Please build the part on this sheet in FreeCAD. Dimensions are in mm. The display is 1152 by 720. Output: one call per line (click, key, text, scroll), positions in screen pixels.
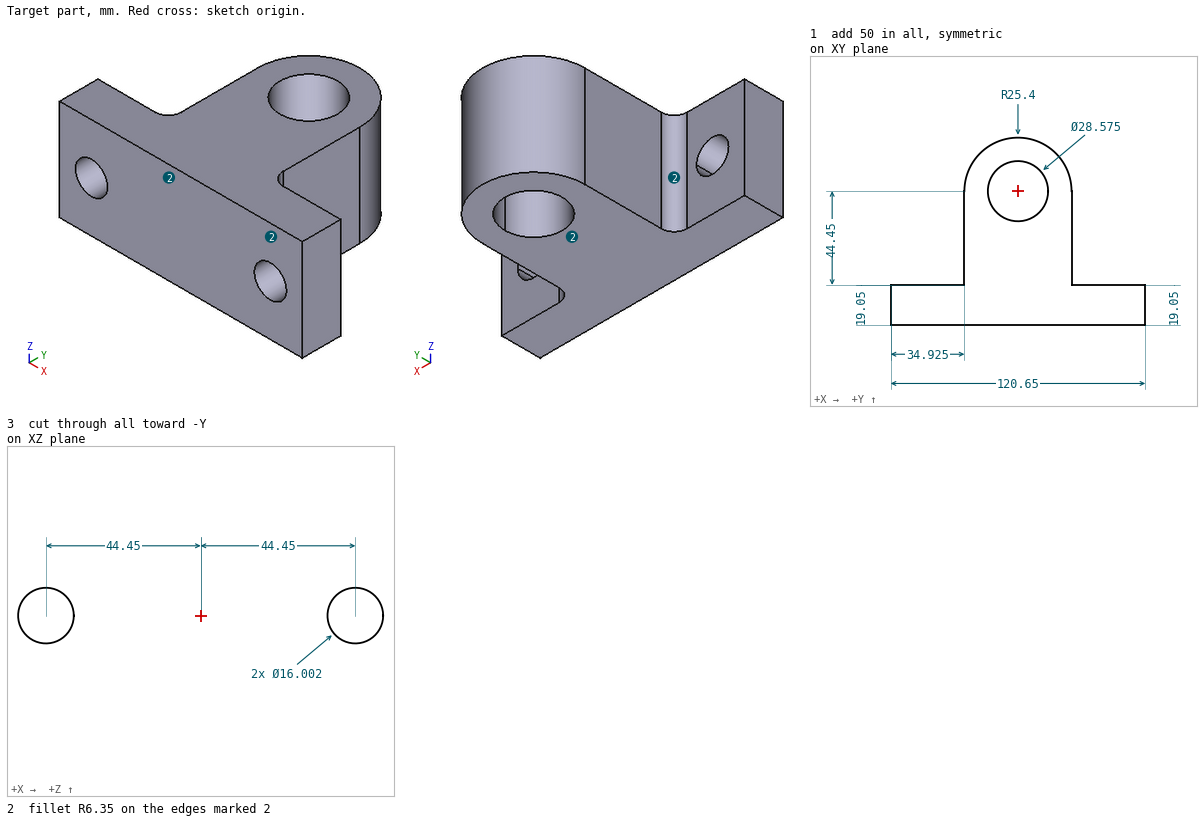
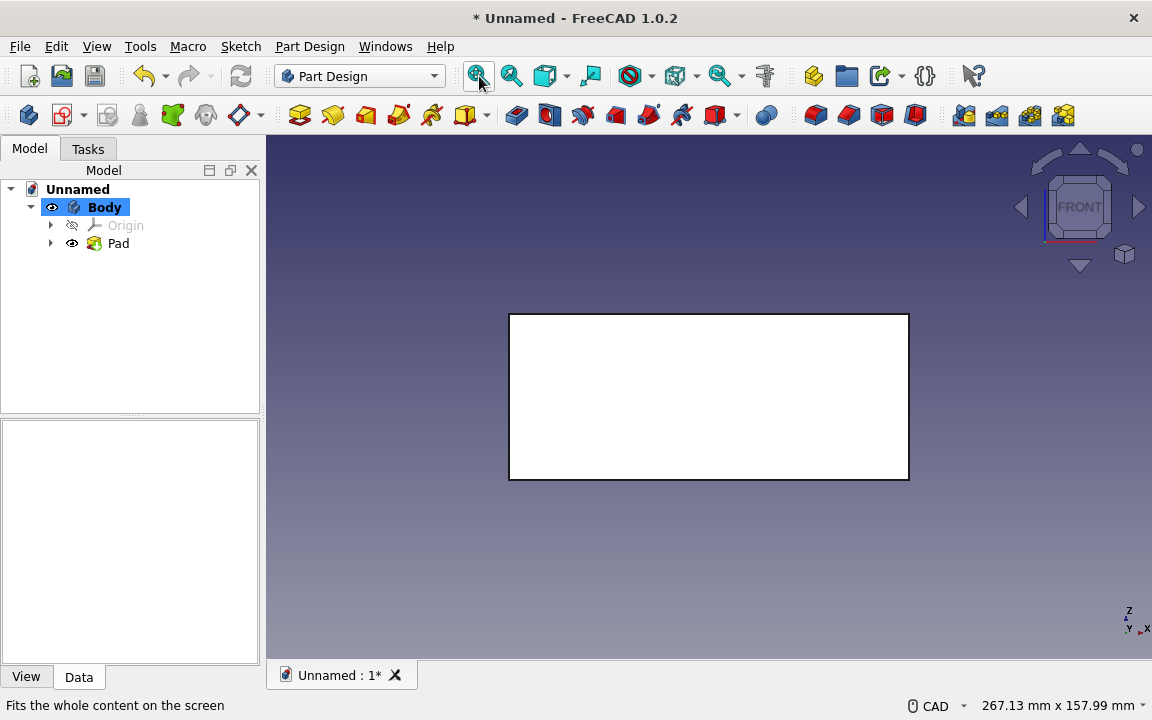
key(3)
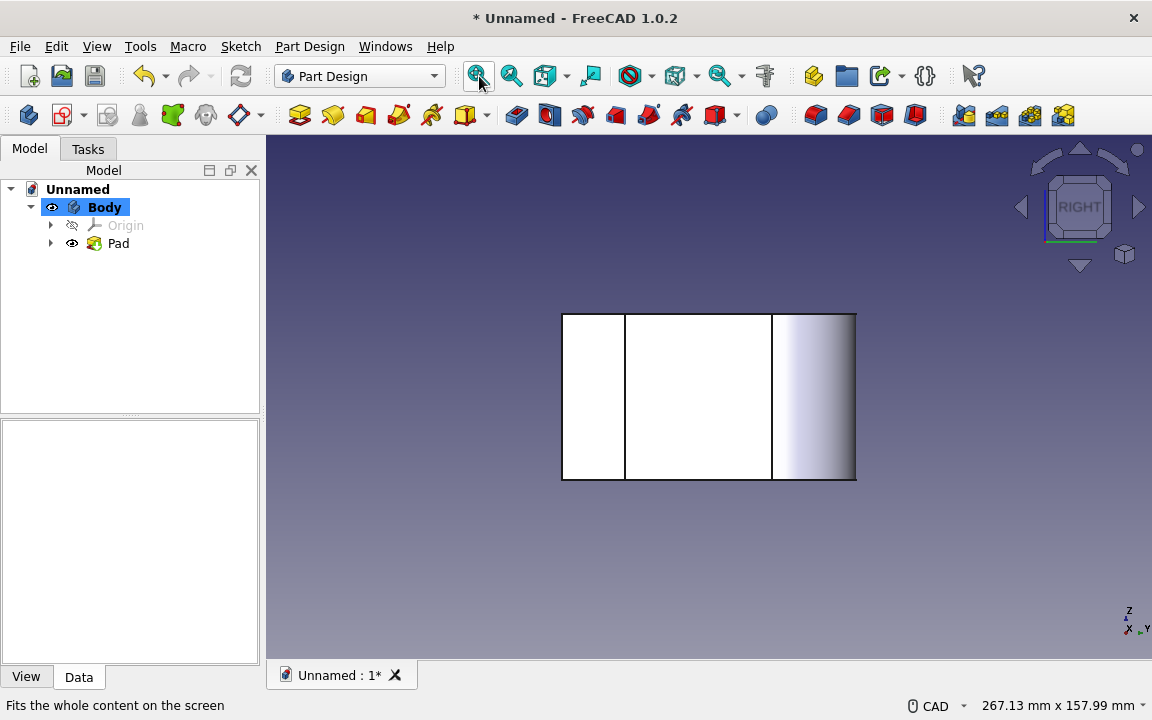
click(479, 76)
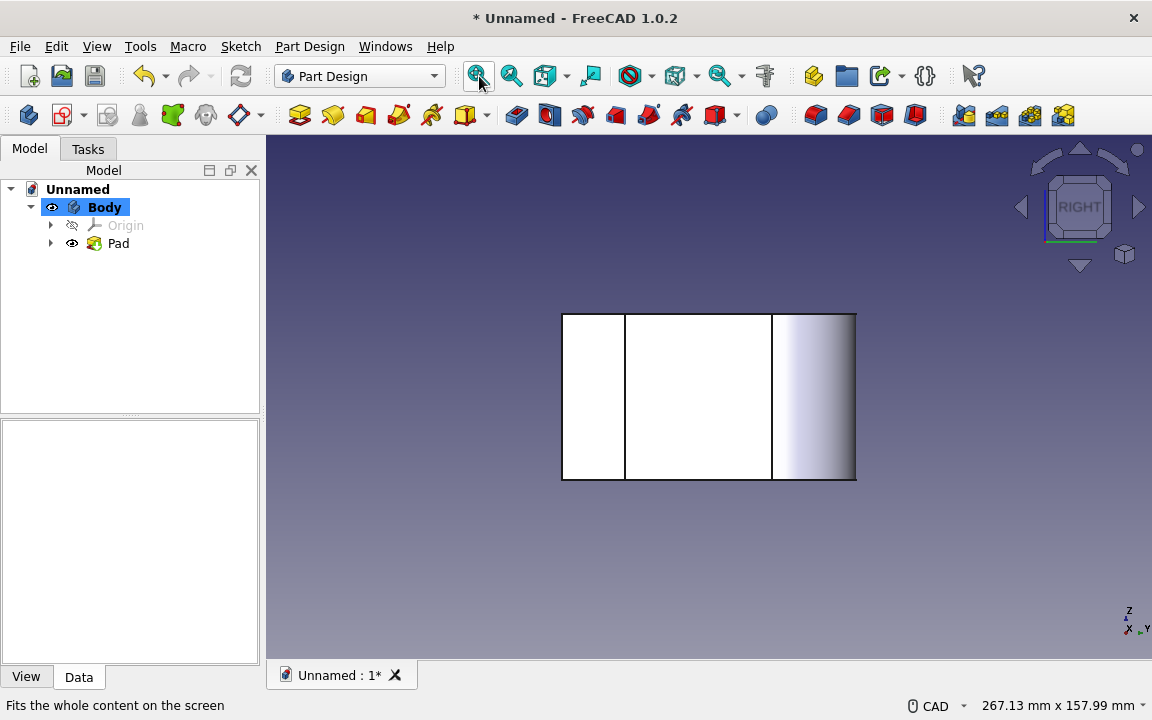
key(5)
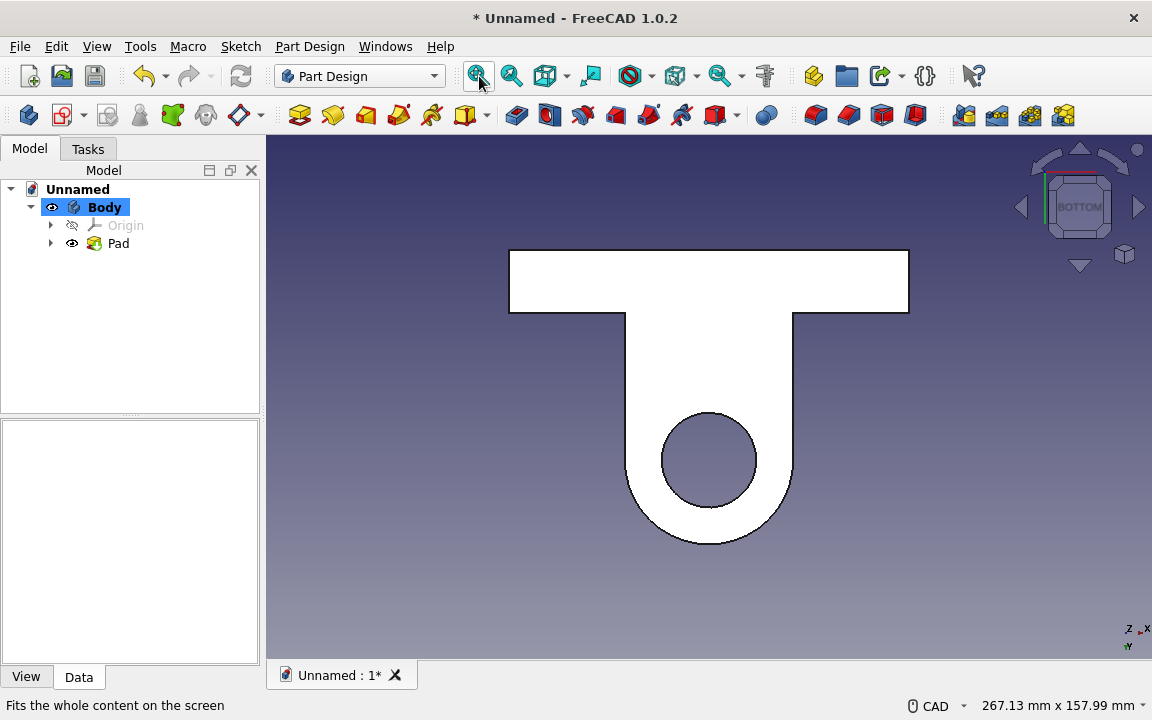
key(4)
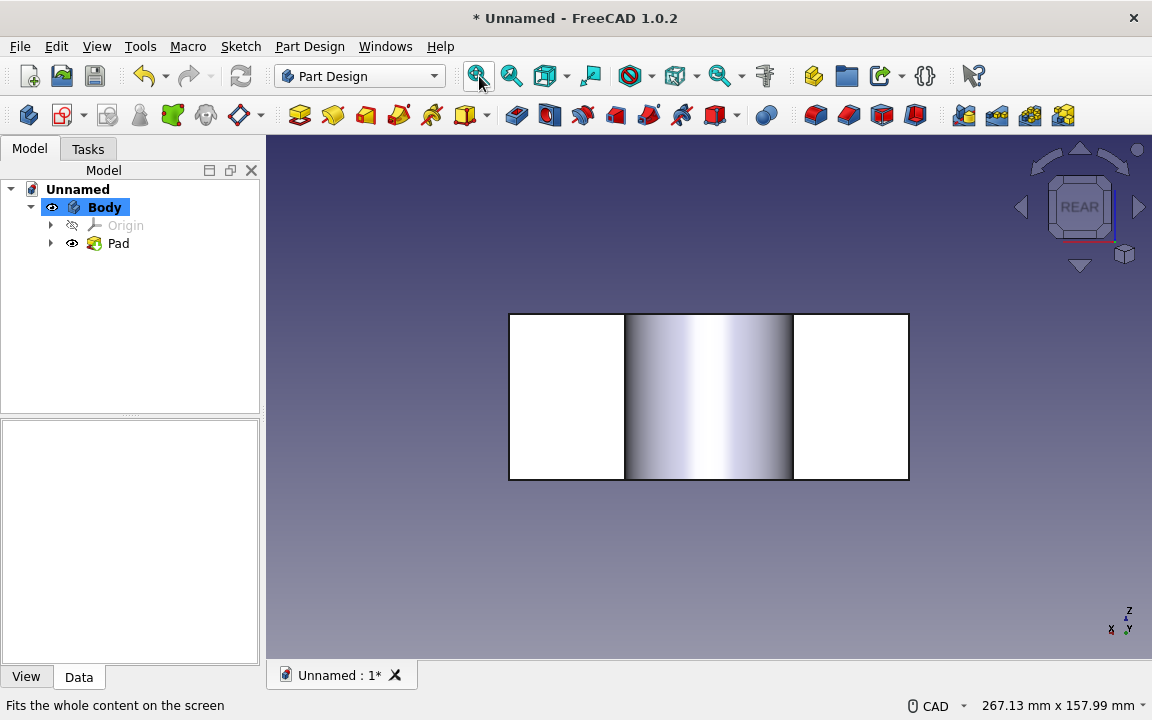
key(6)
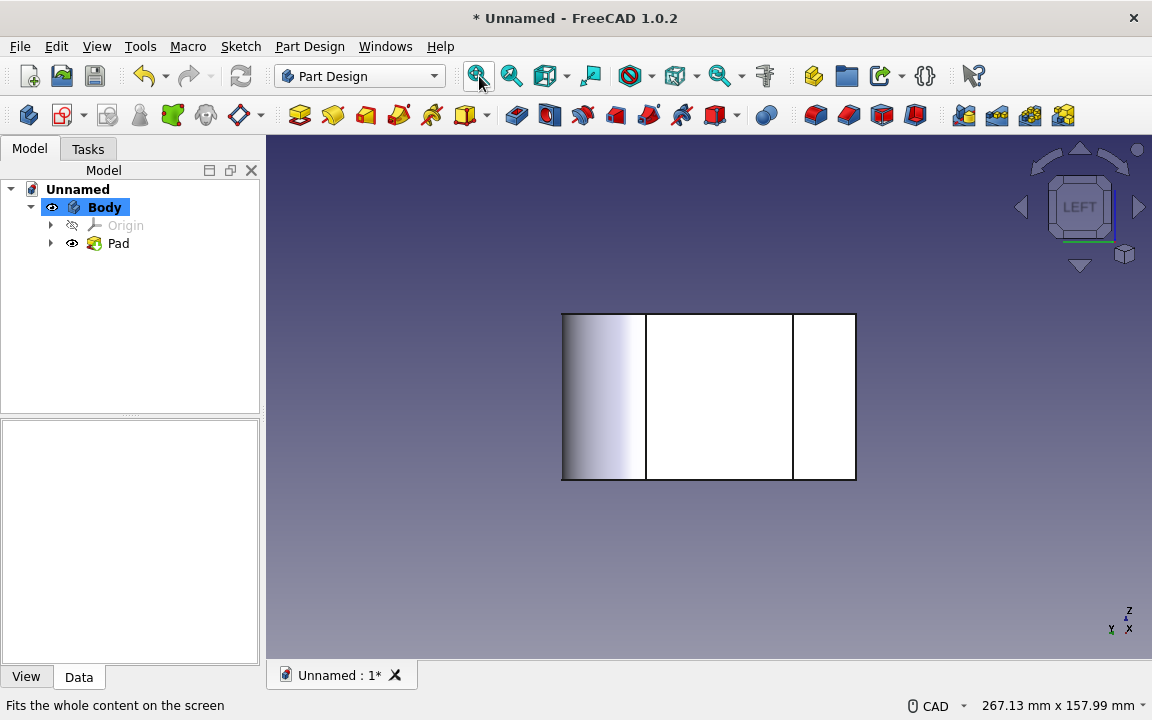
click(479, 76)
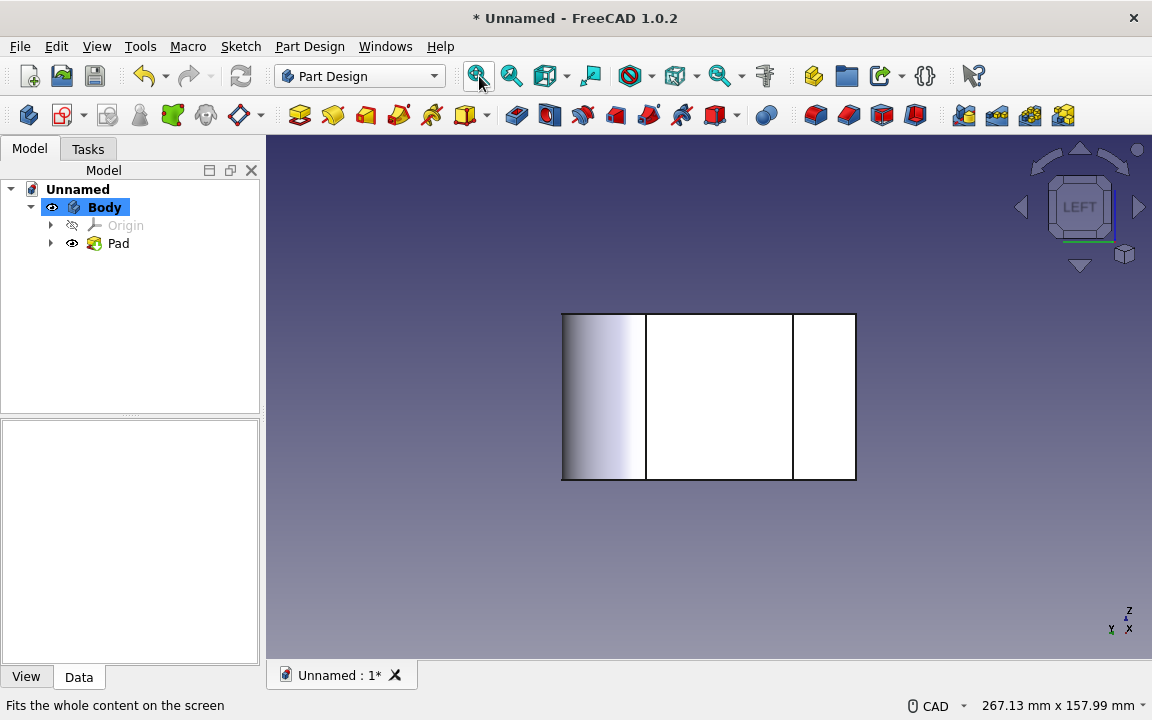
key(v)
key(3)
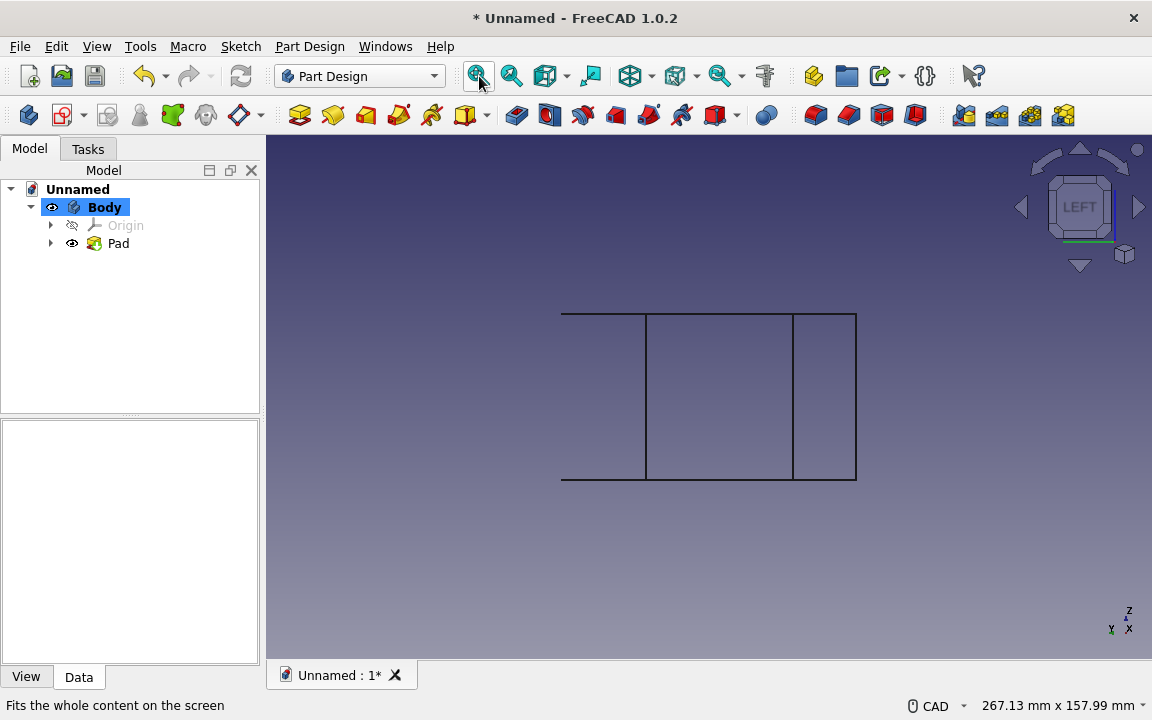
key(0)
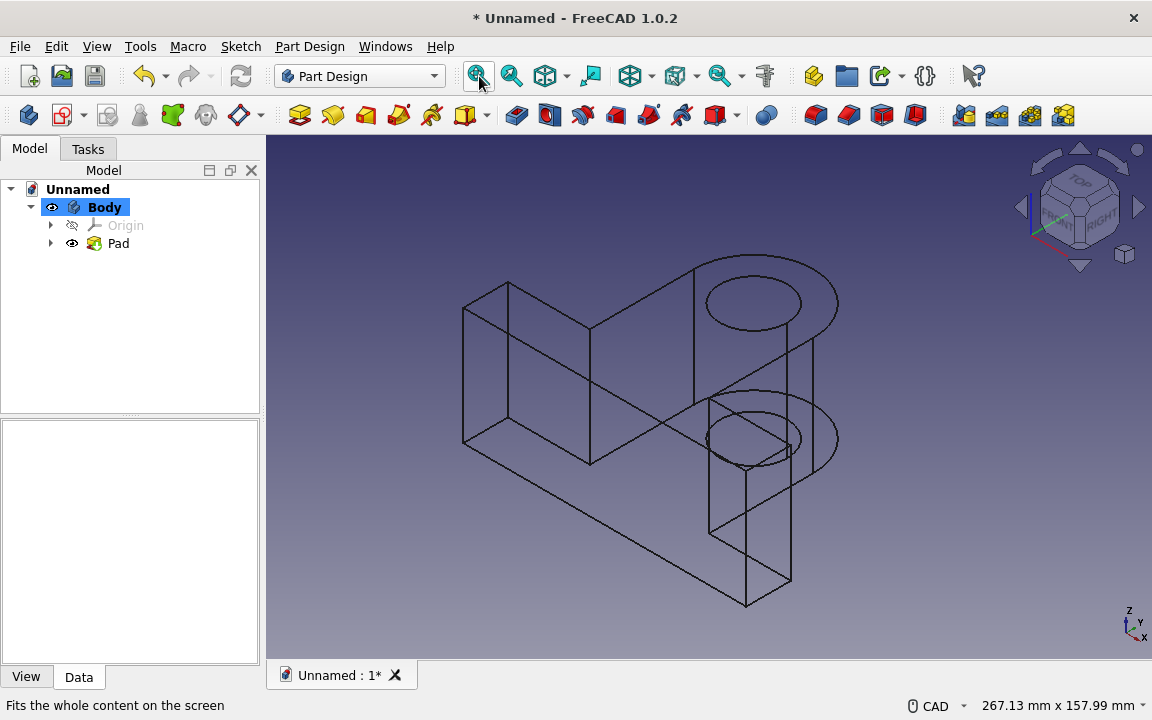
click(709, 465)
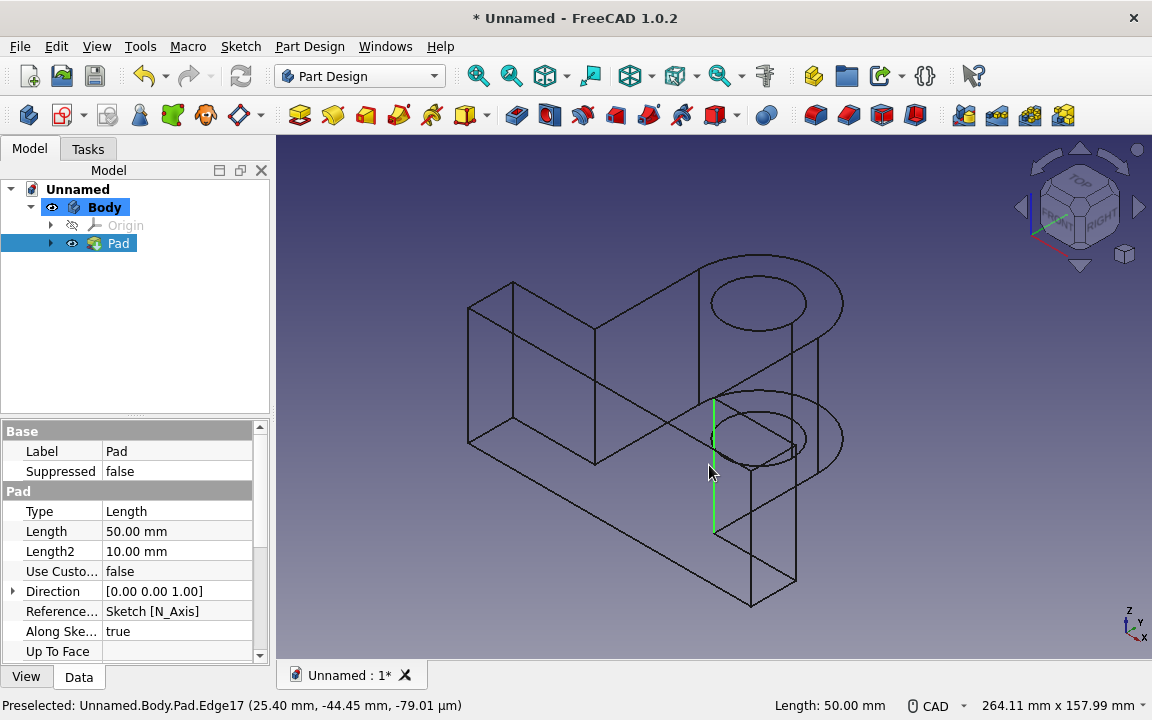
click(595, 396, ctrl)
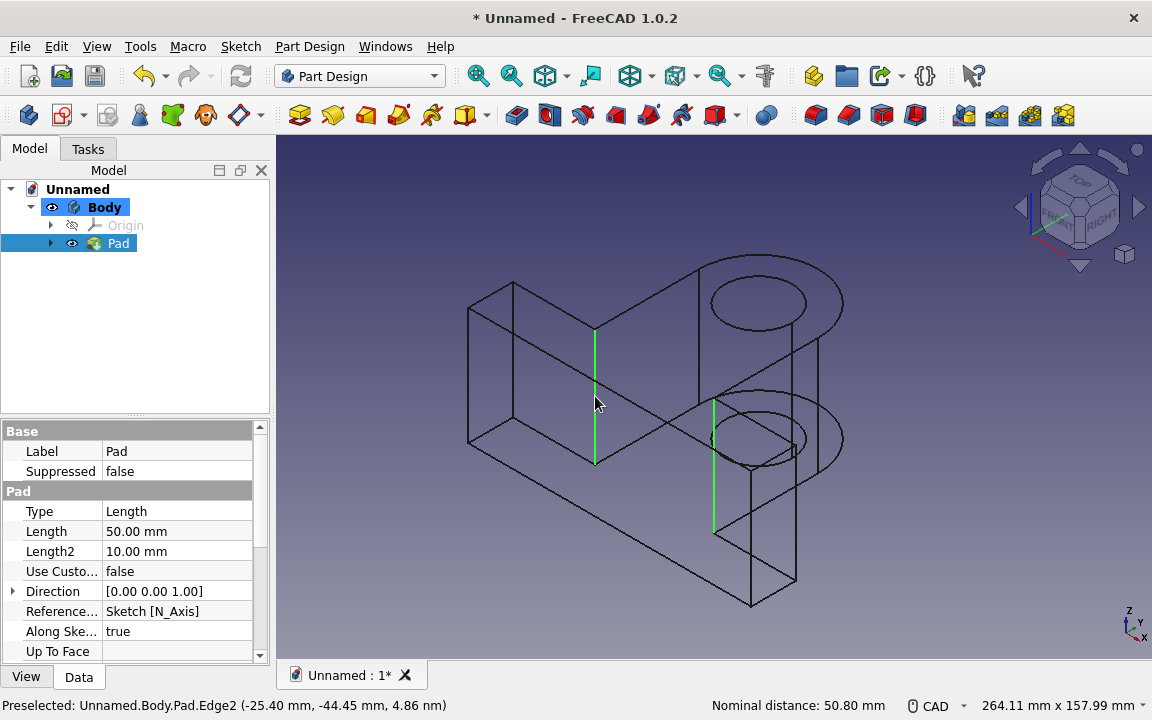
key(v)
key(1)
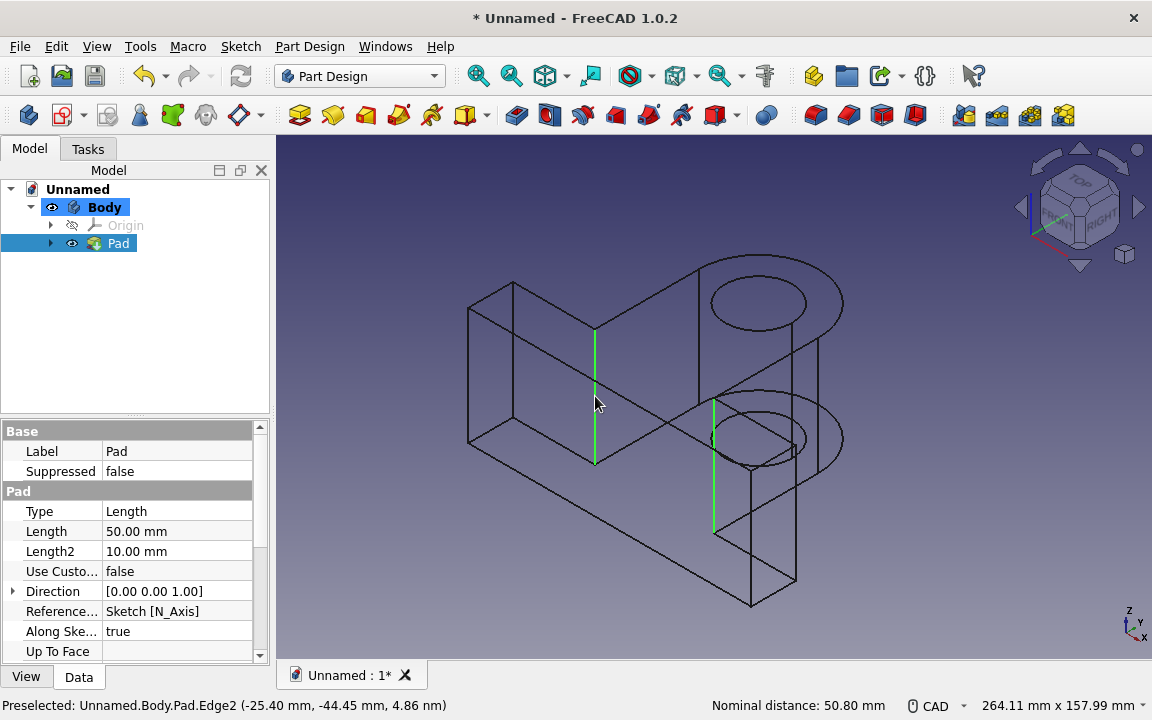
click(816, 116)